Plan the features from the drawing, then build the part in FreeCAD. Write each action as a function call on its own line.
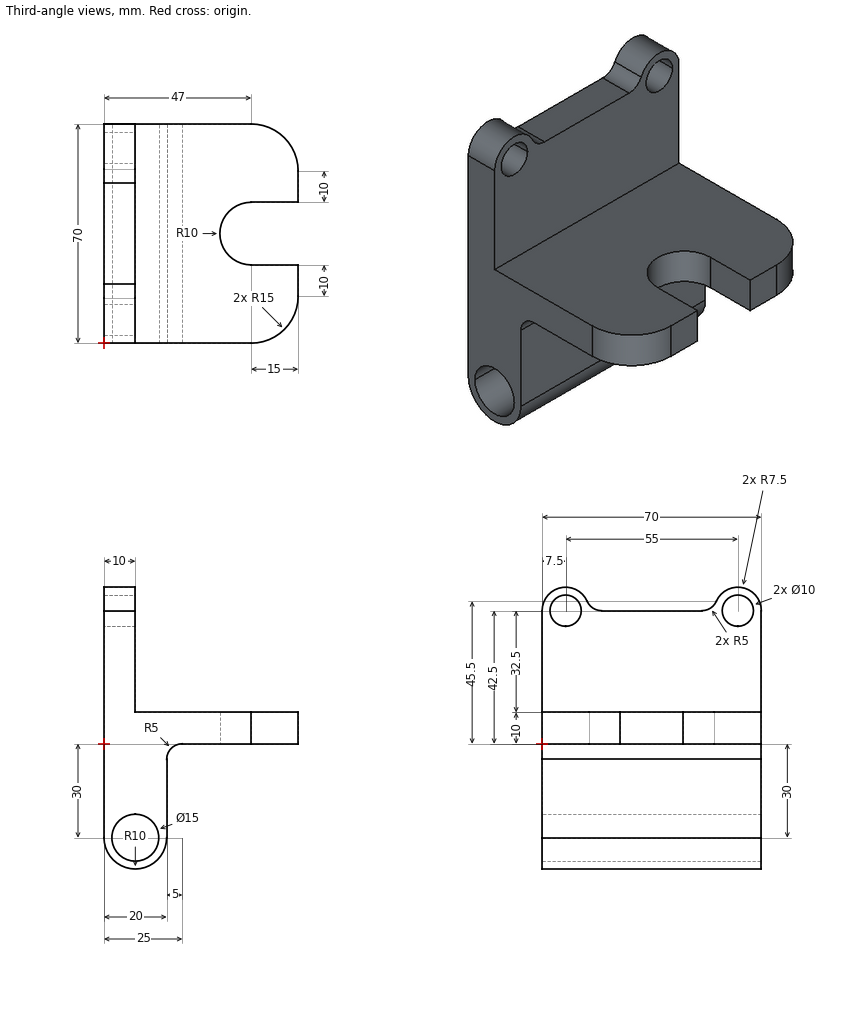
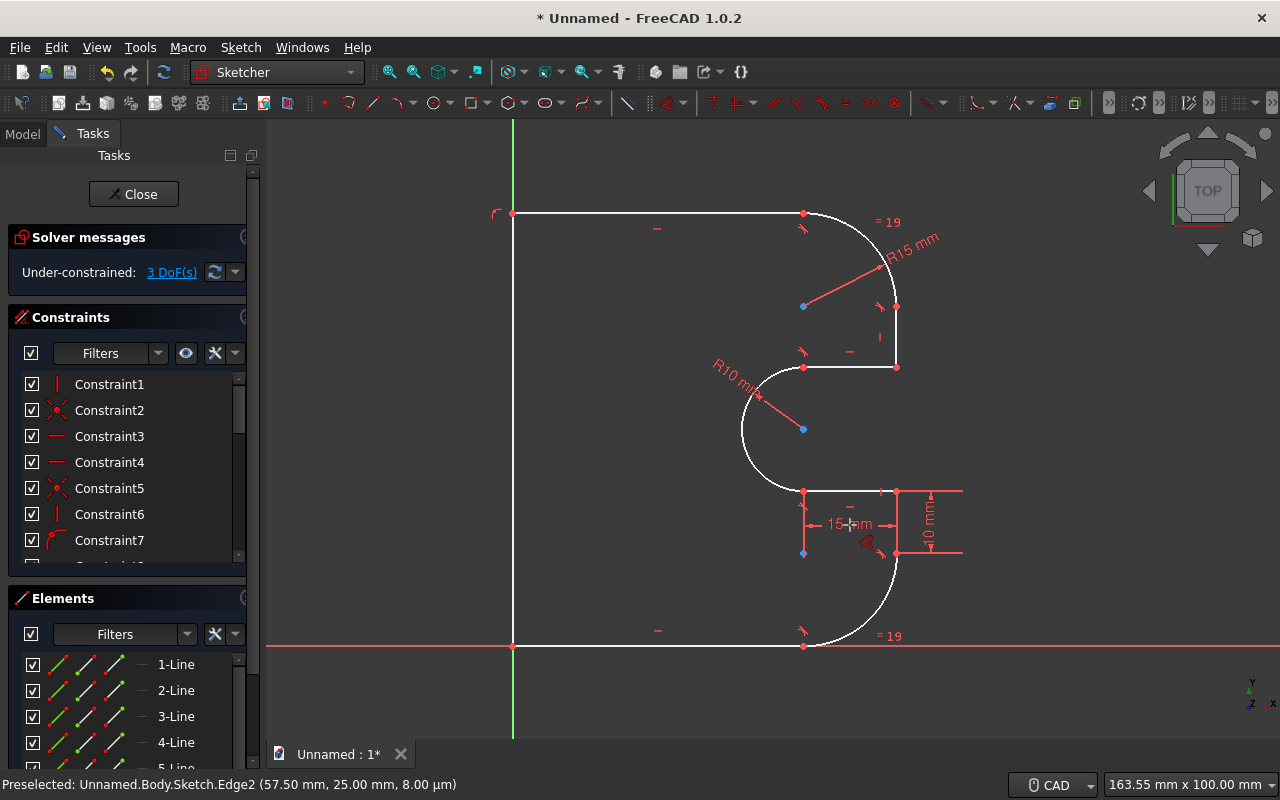
click(832, 367)
click(850, 333)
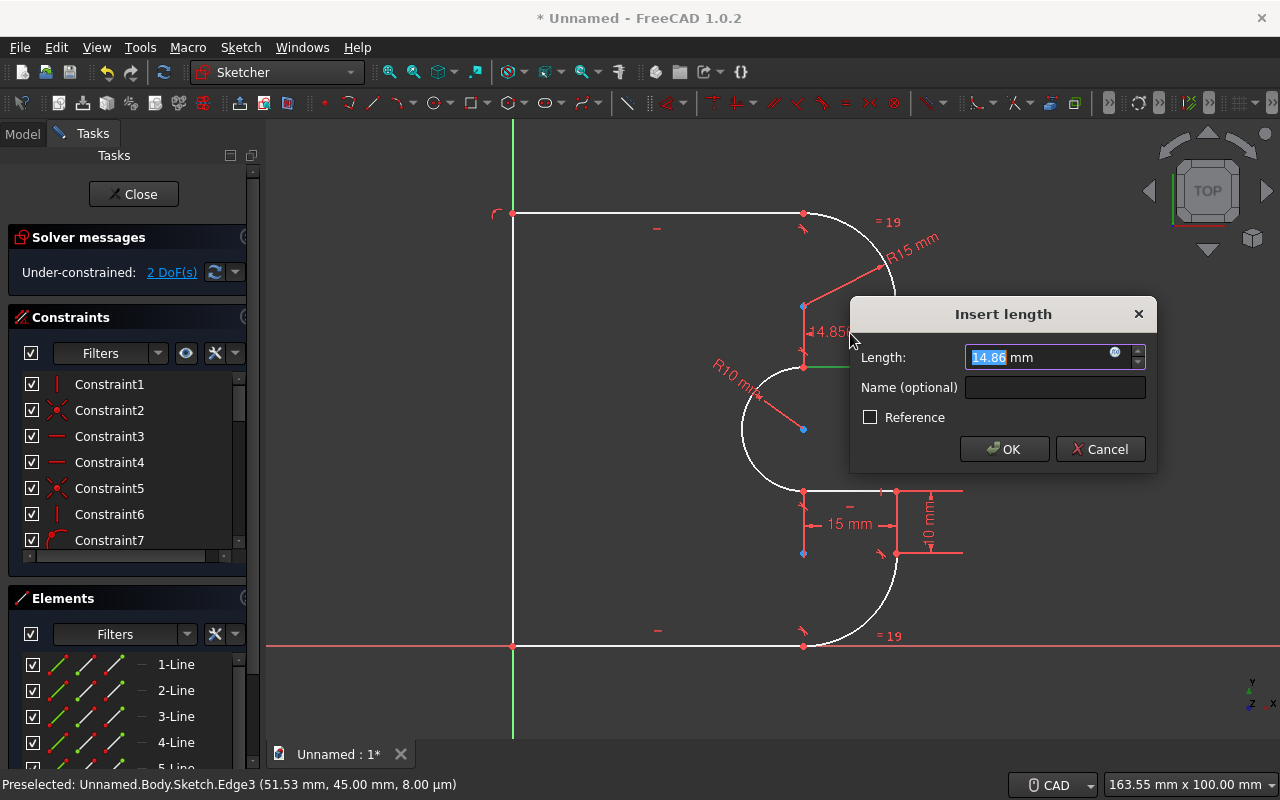
text(15)
key(Return)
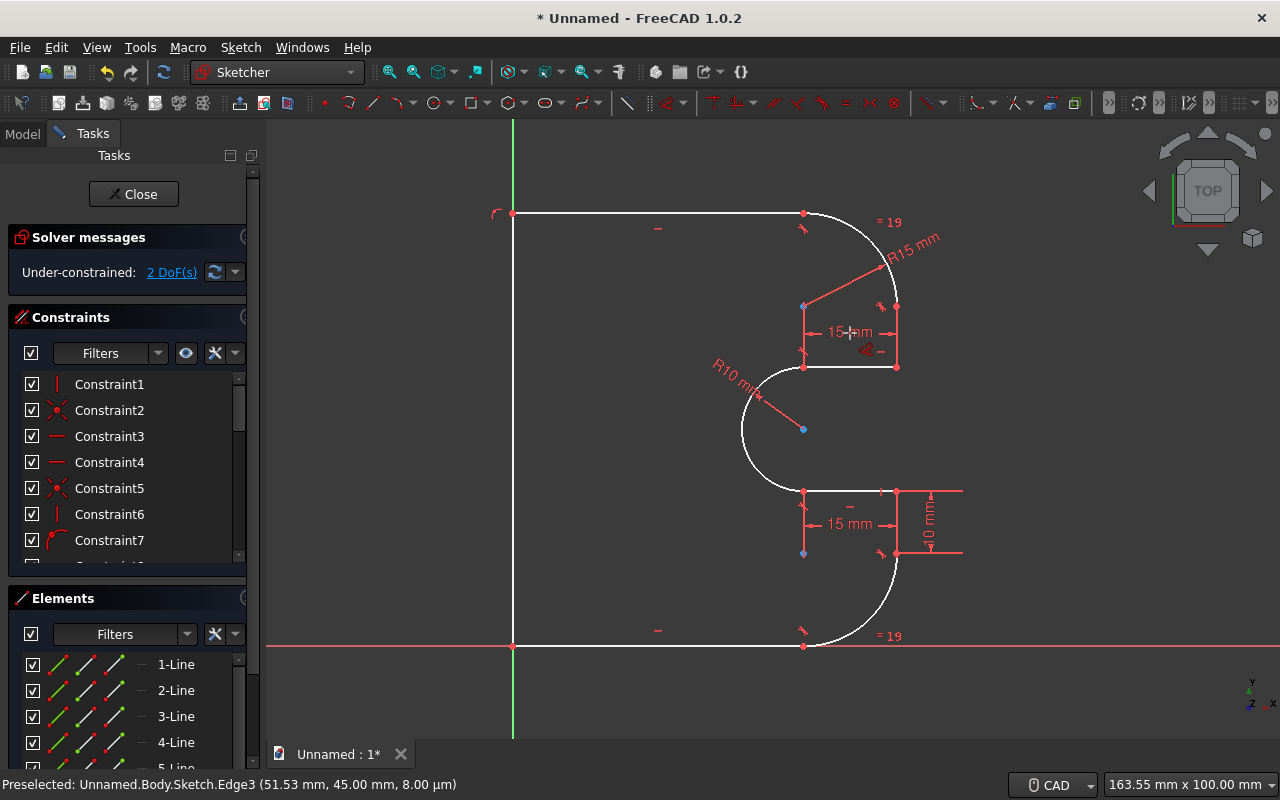
click(897, 349)
click(931, 337)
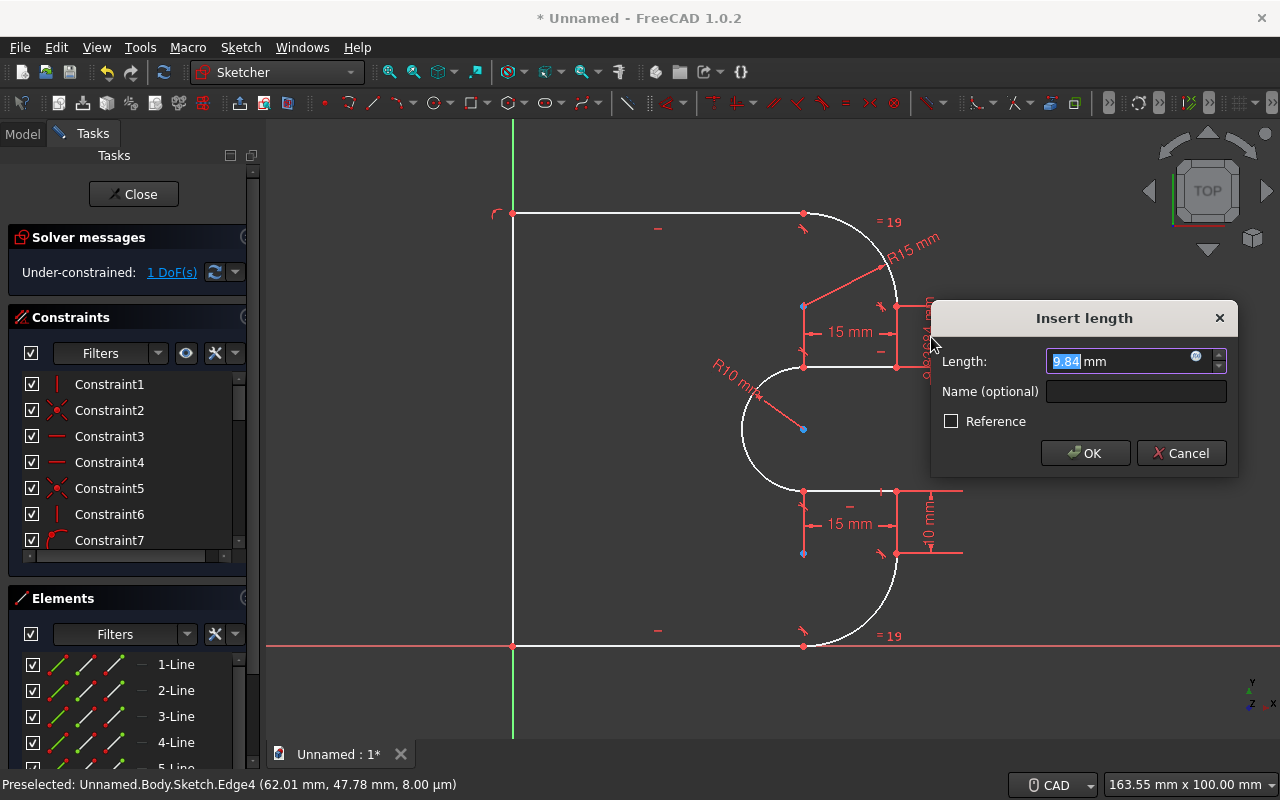
text(10)
key(Return)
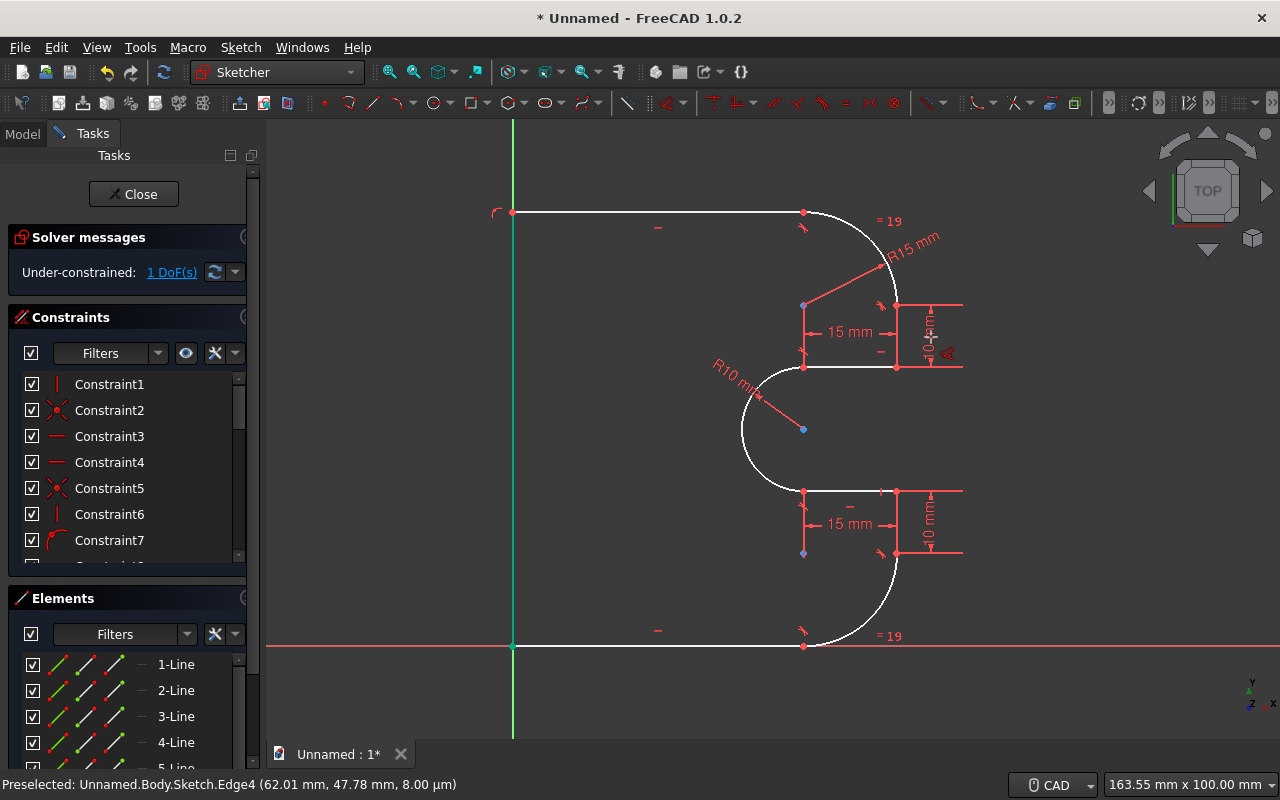
click(717, 212)
click(658, 178)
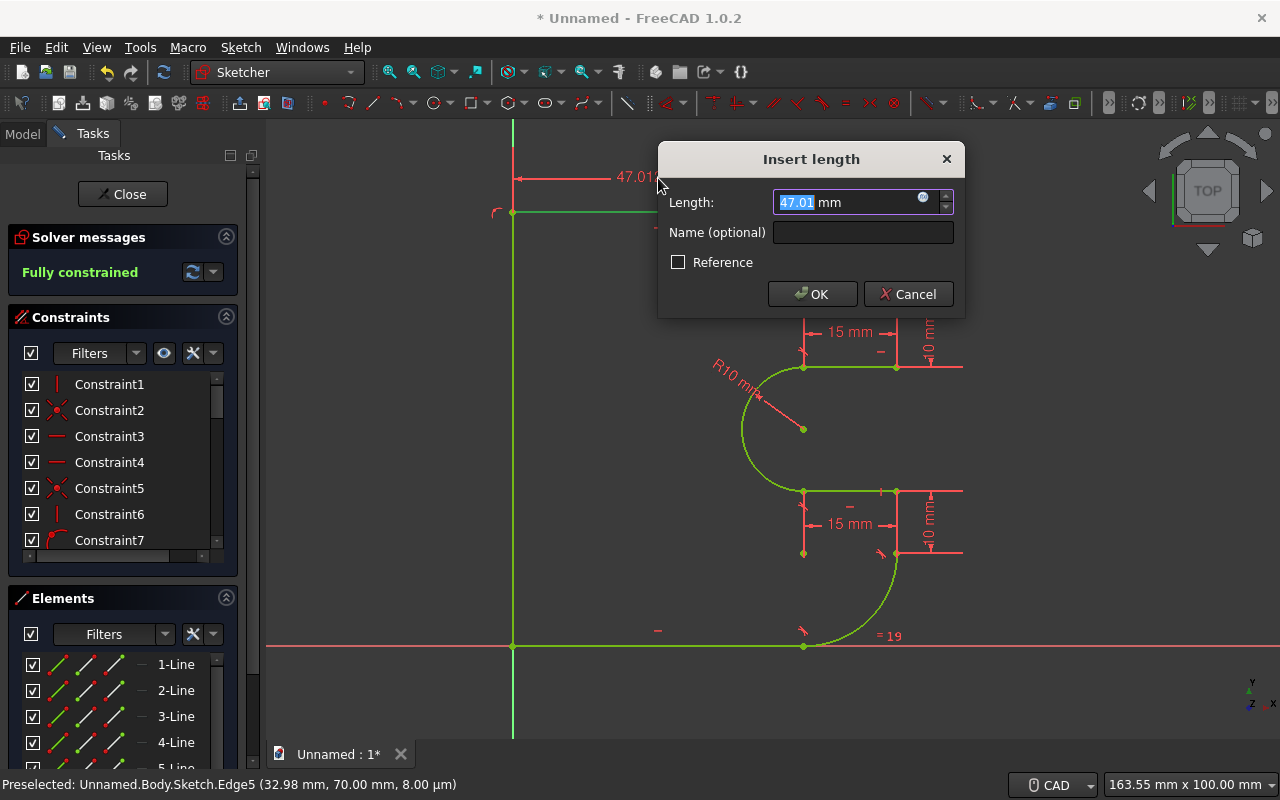
text(47)
key(Return)
key(Escape)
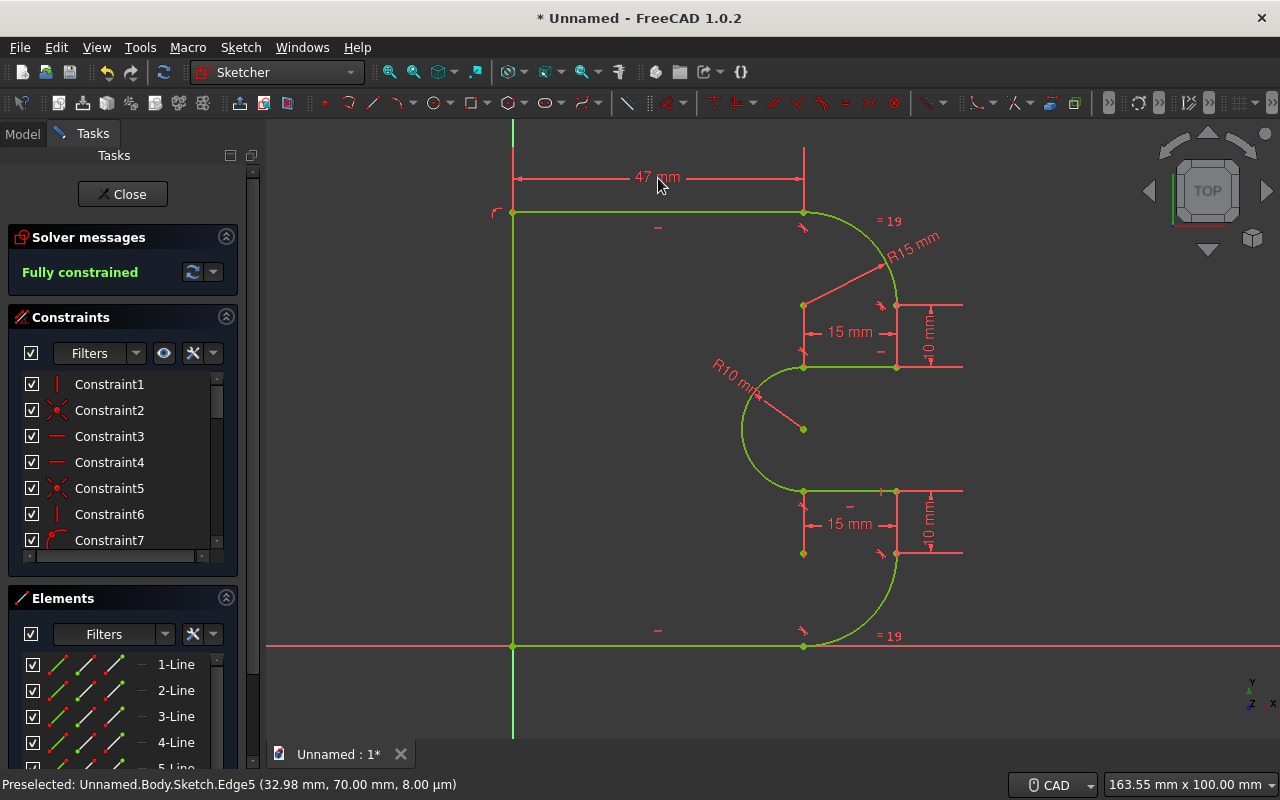
click(123, 194)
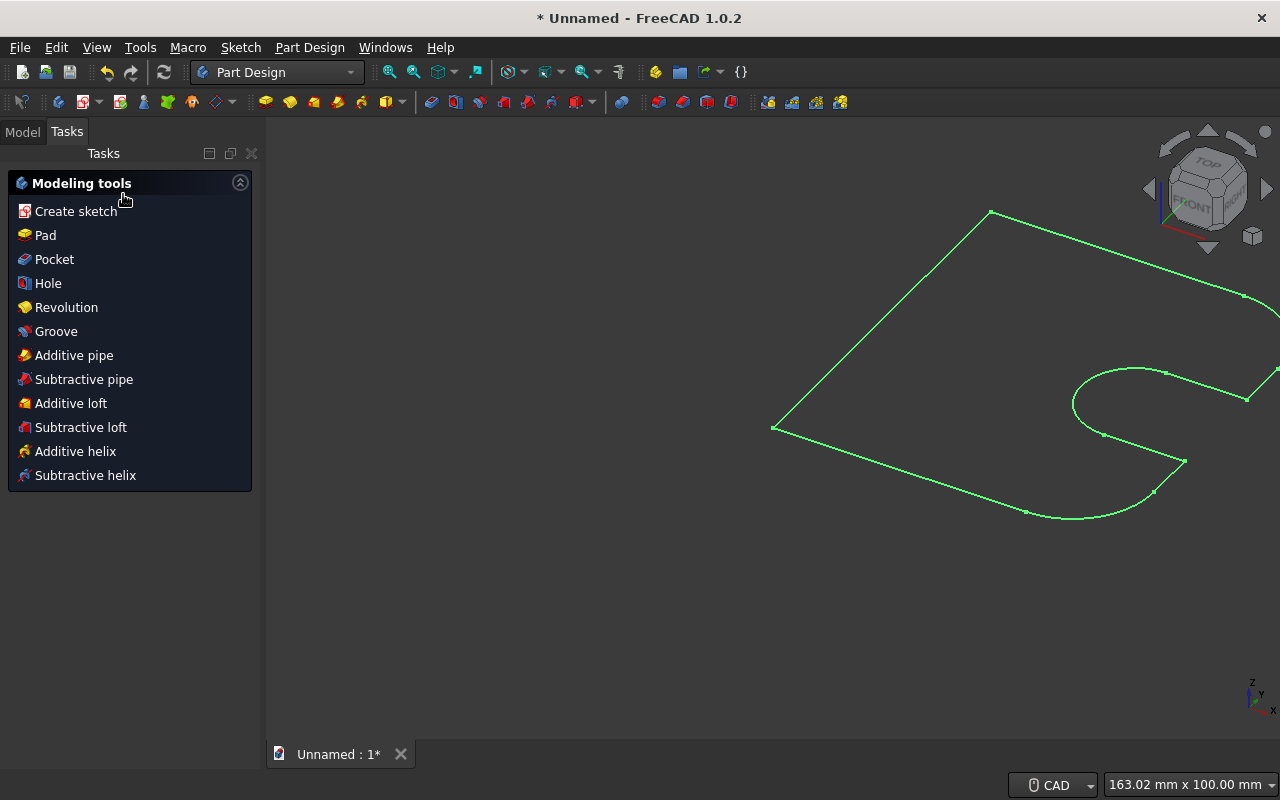
click(266, 102)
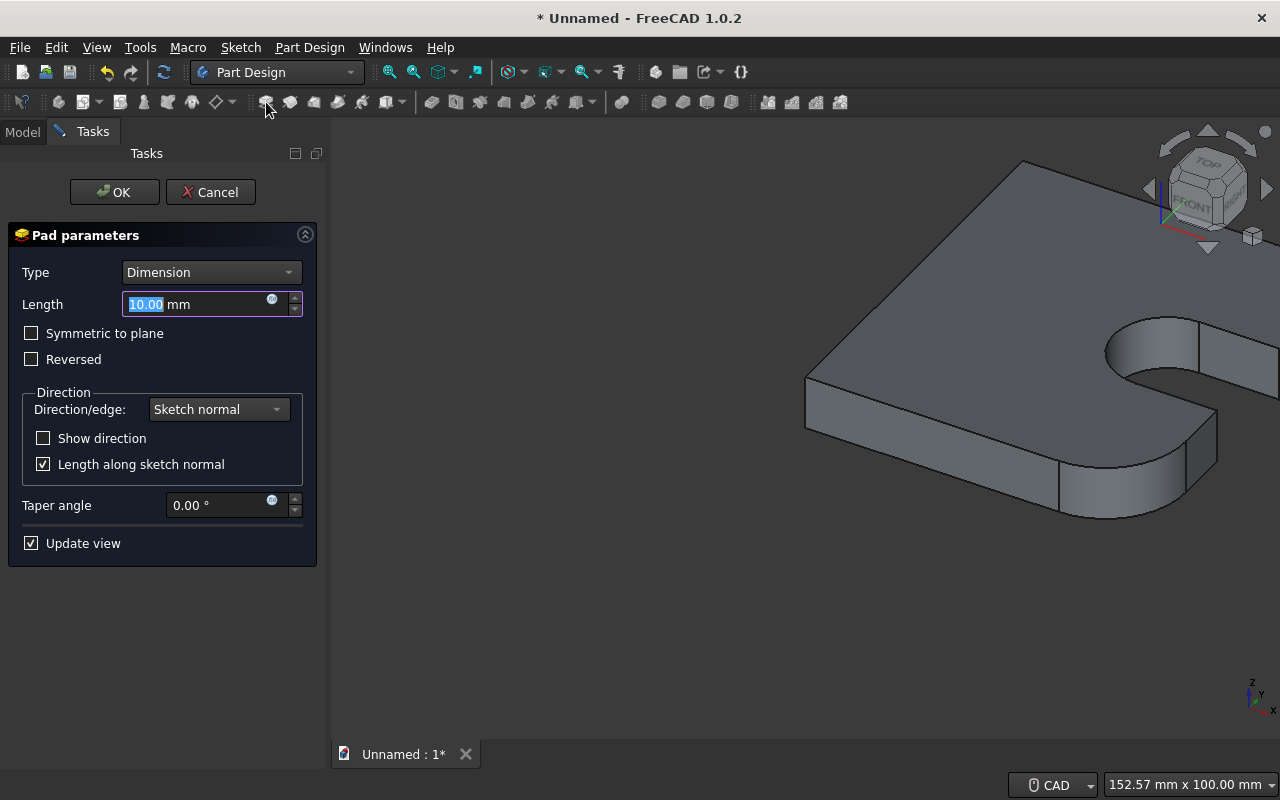
text(10)
key(Tab)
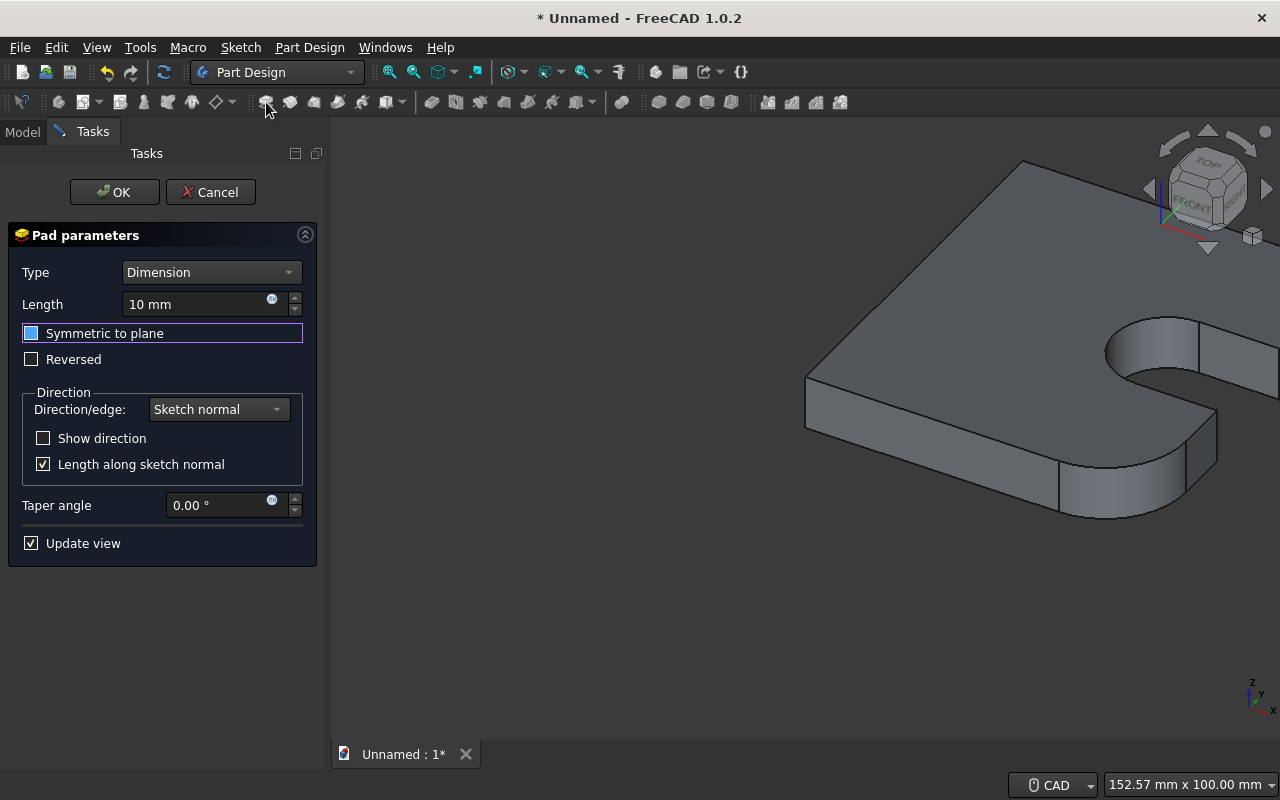
click(115, 192)